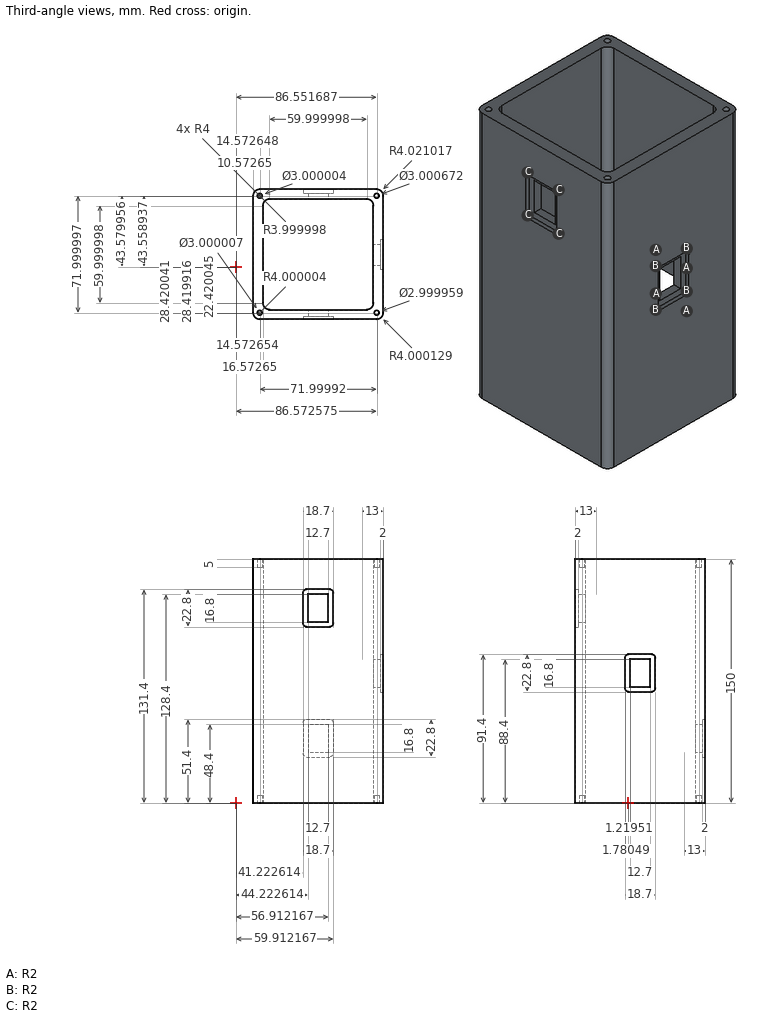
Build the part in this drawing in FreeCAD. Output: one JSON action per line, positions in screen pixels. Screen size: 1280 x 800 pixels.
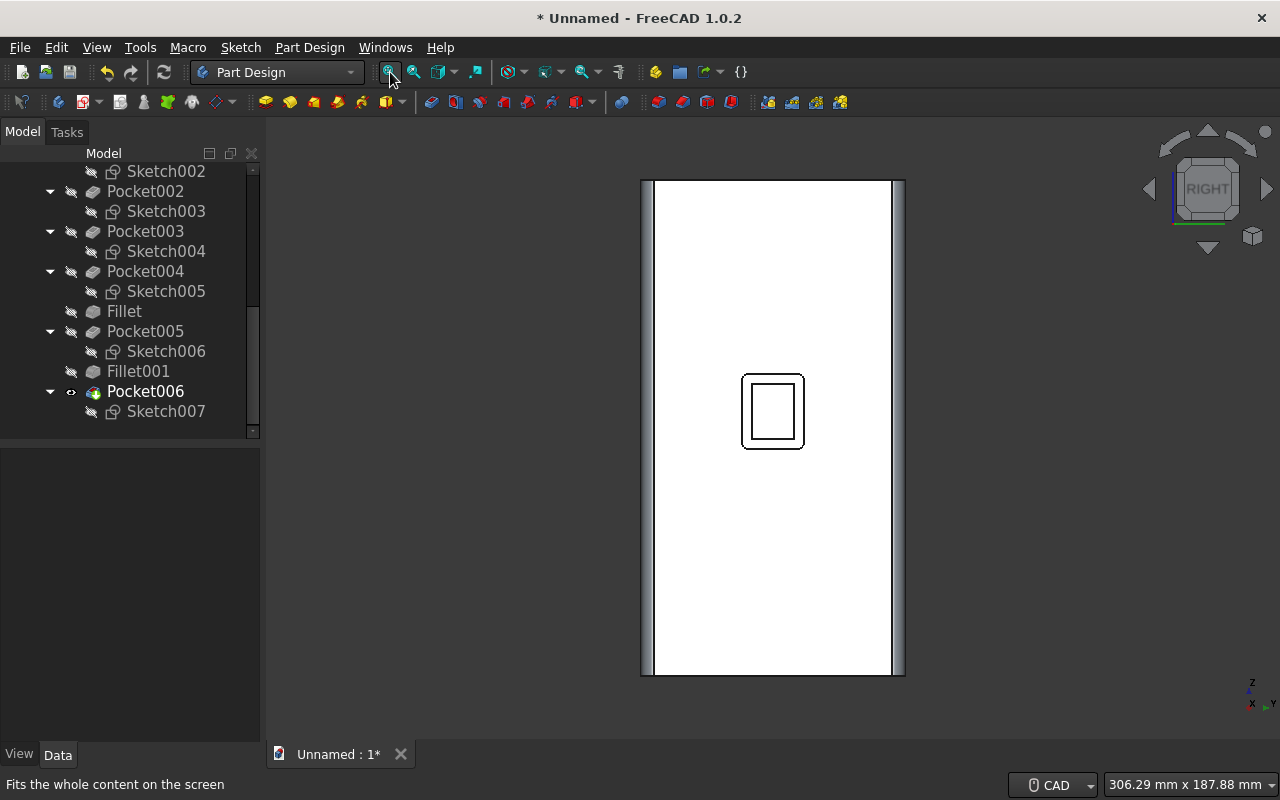
{"action": "scroll", "coordinate": [644, 316], "scroll_direction": "up", "scroll_amount": 9}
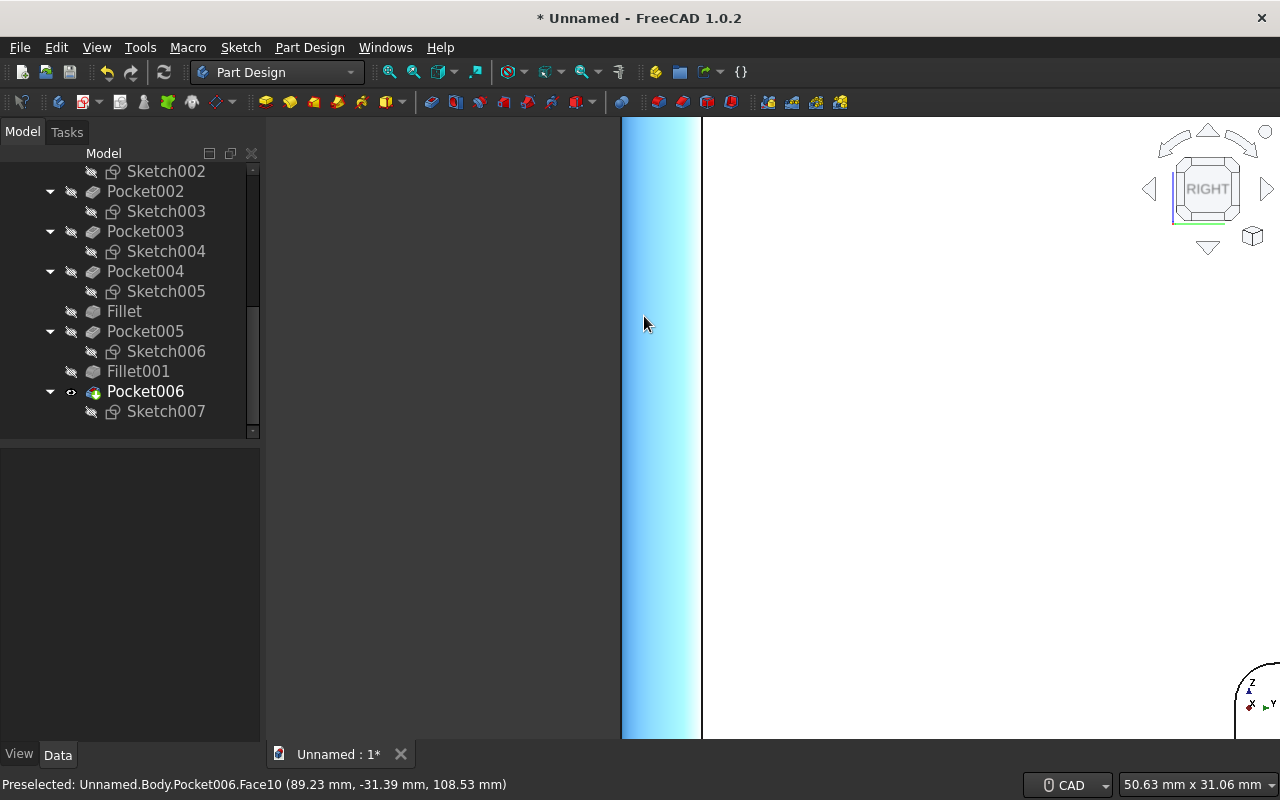
{"action": "left_click", "coordinate": [390, 72]}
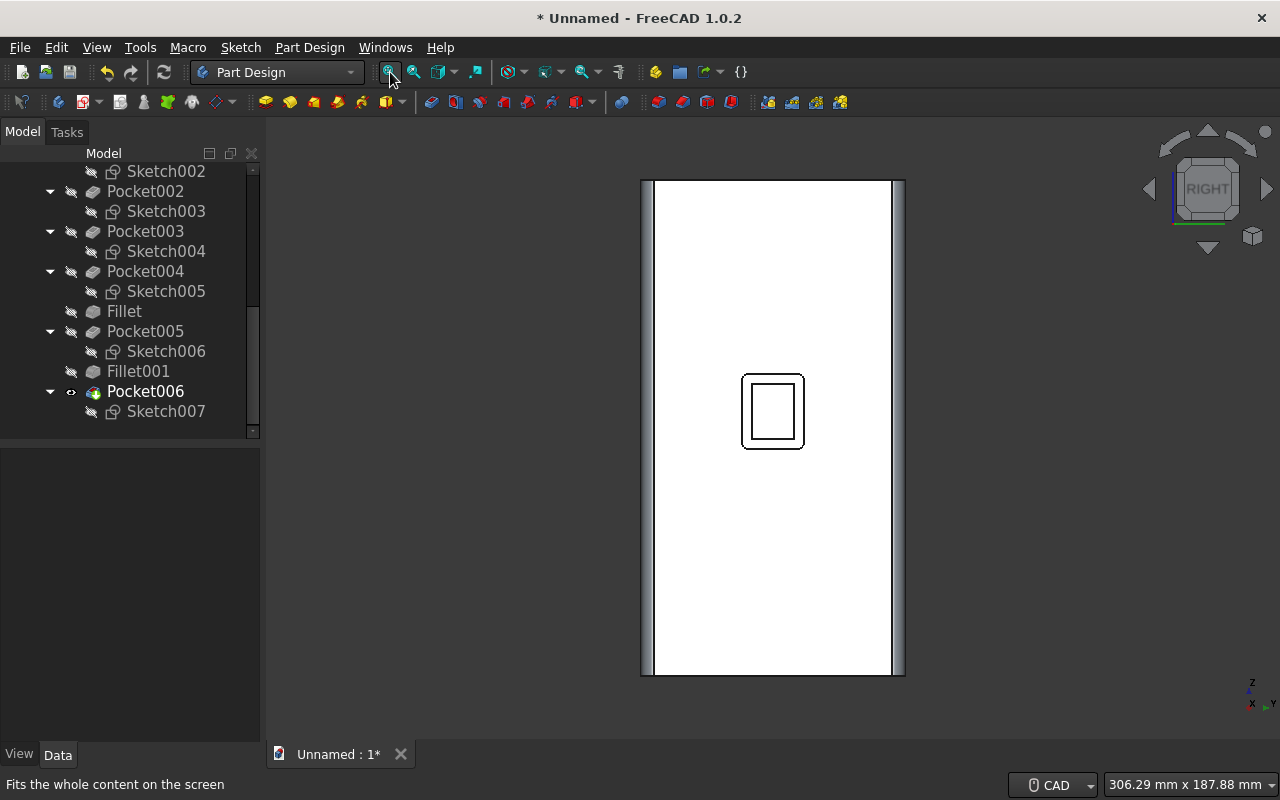
{"action": "key", "text": "5"}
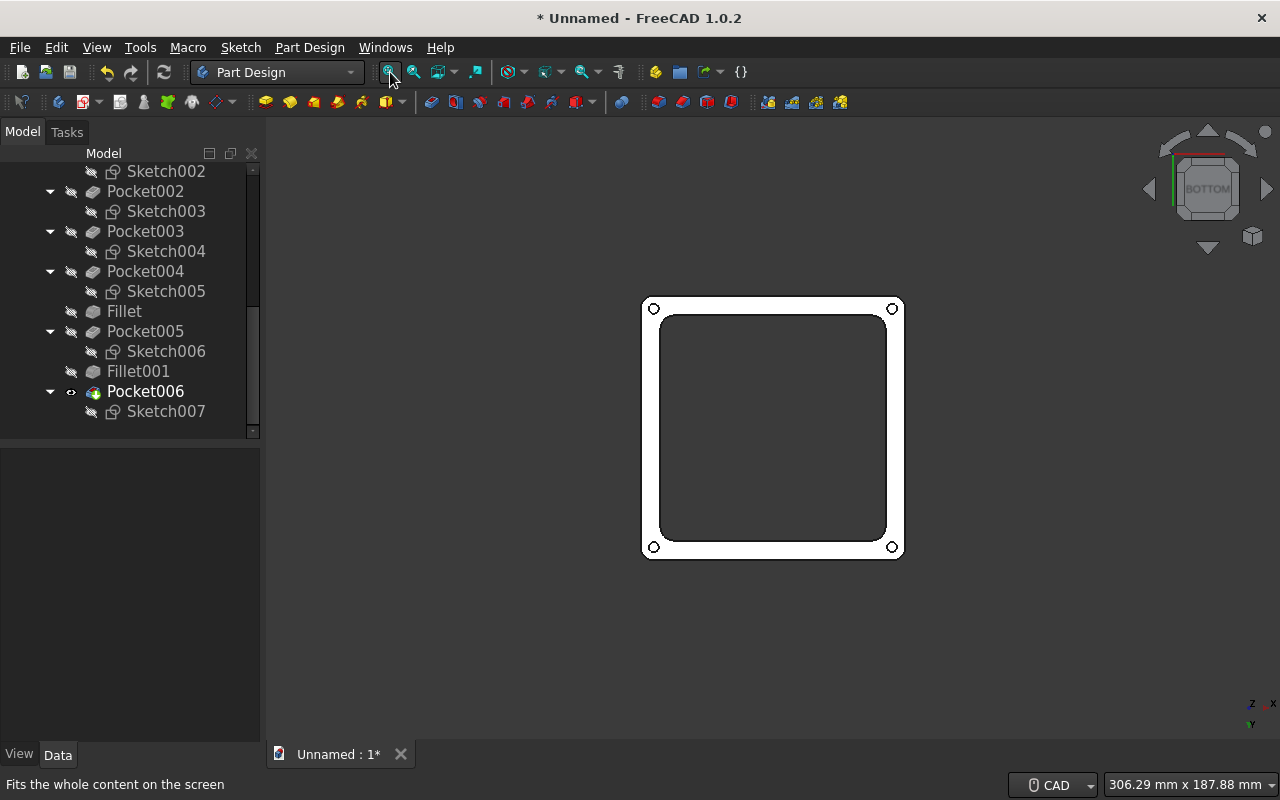
{"action": "left_click", "coordinate": [390, 72]}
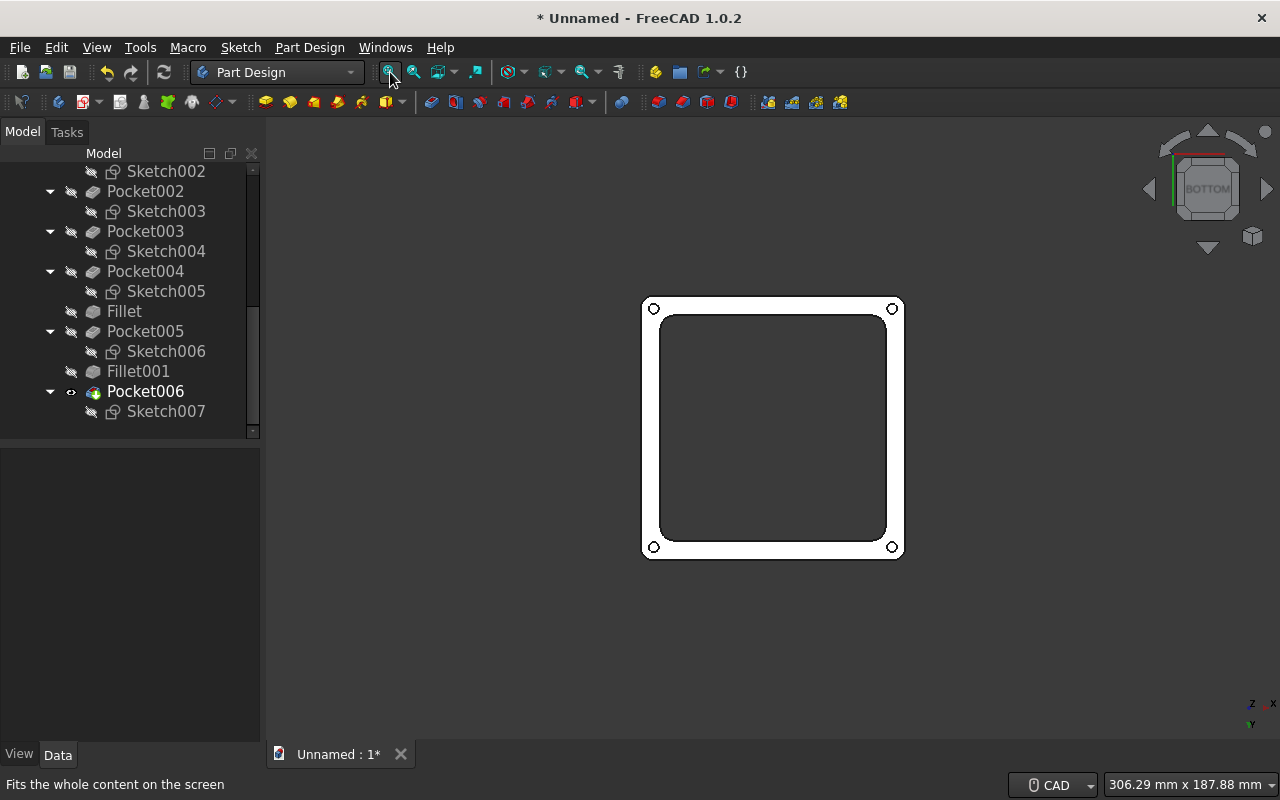
{"action": "scroll", "coordinate": [742, 298], "scroll_direction": "up", "scroll_amount": 9}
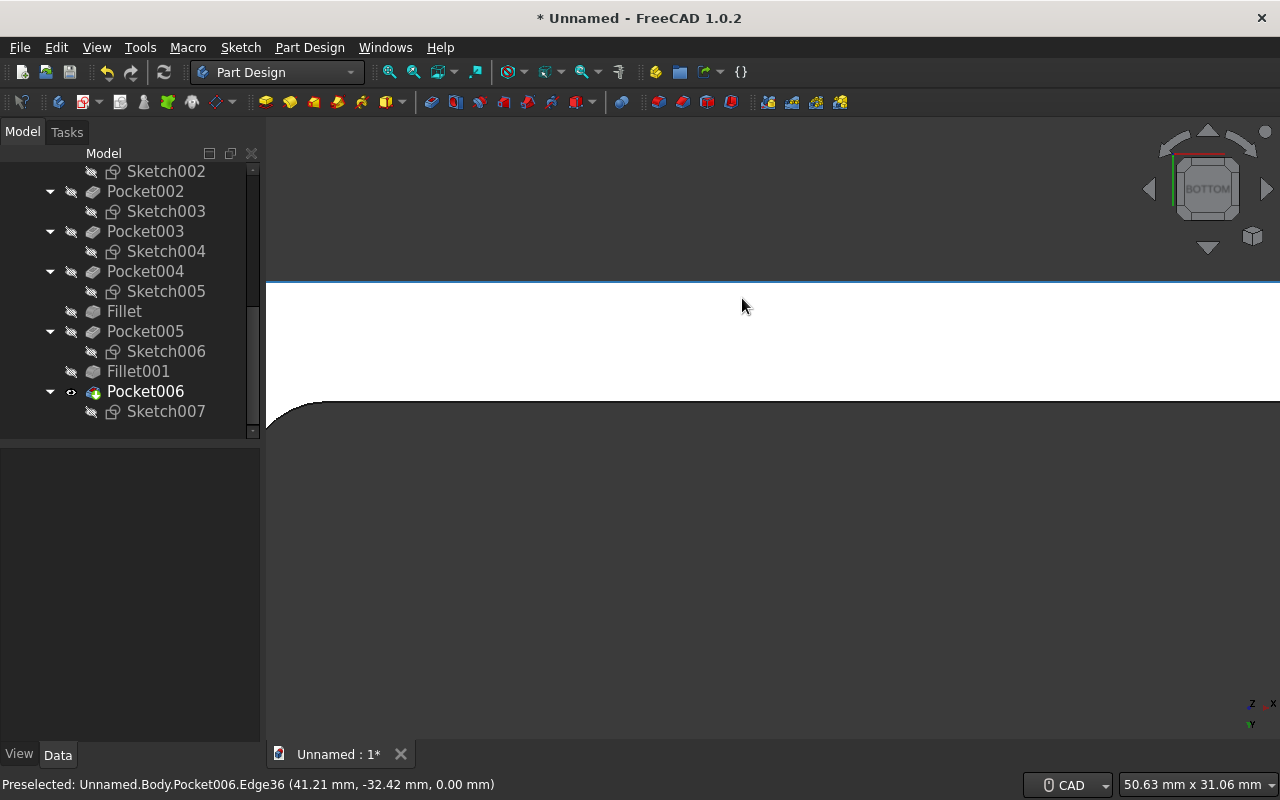
{"action": "left_click", "coordinate": [390, 72]}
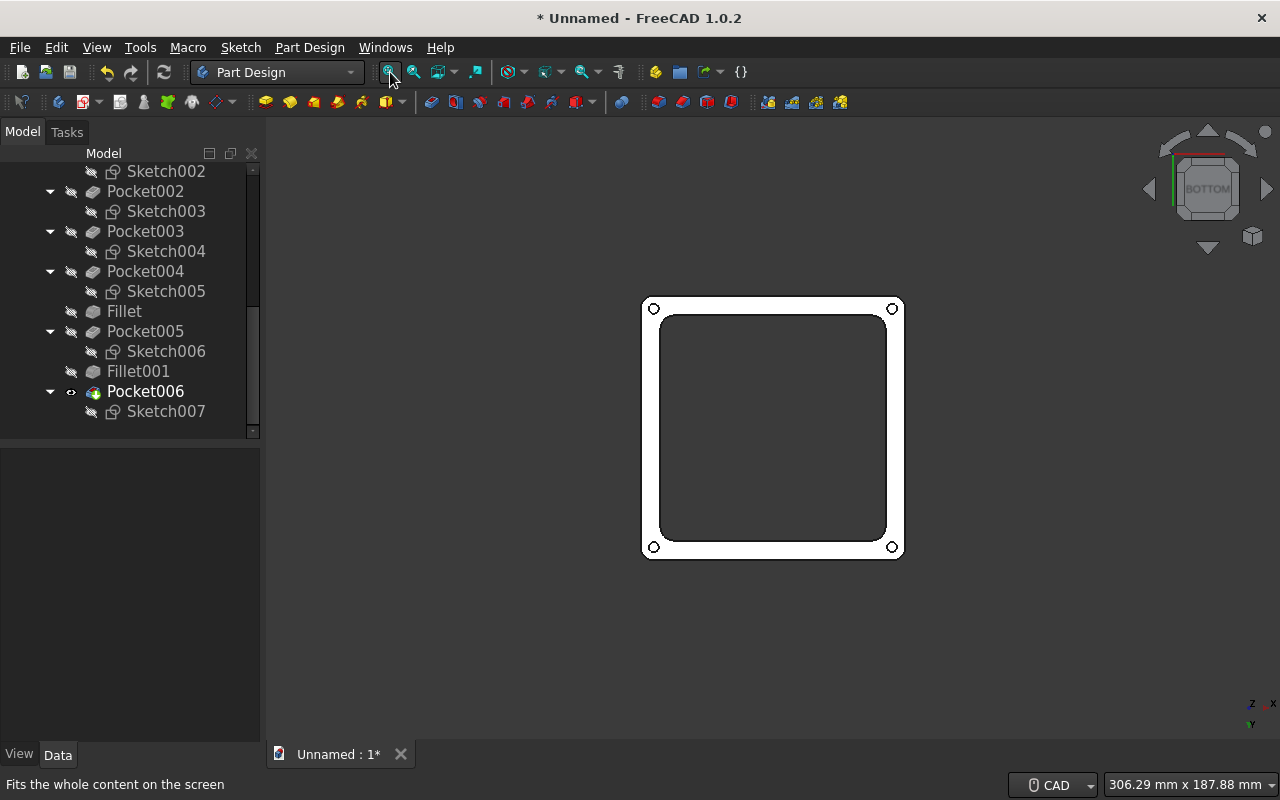
{"action": "key", "text": "4"}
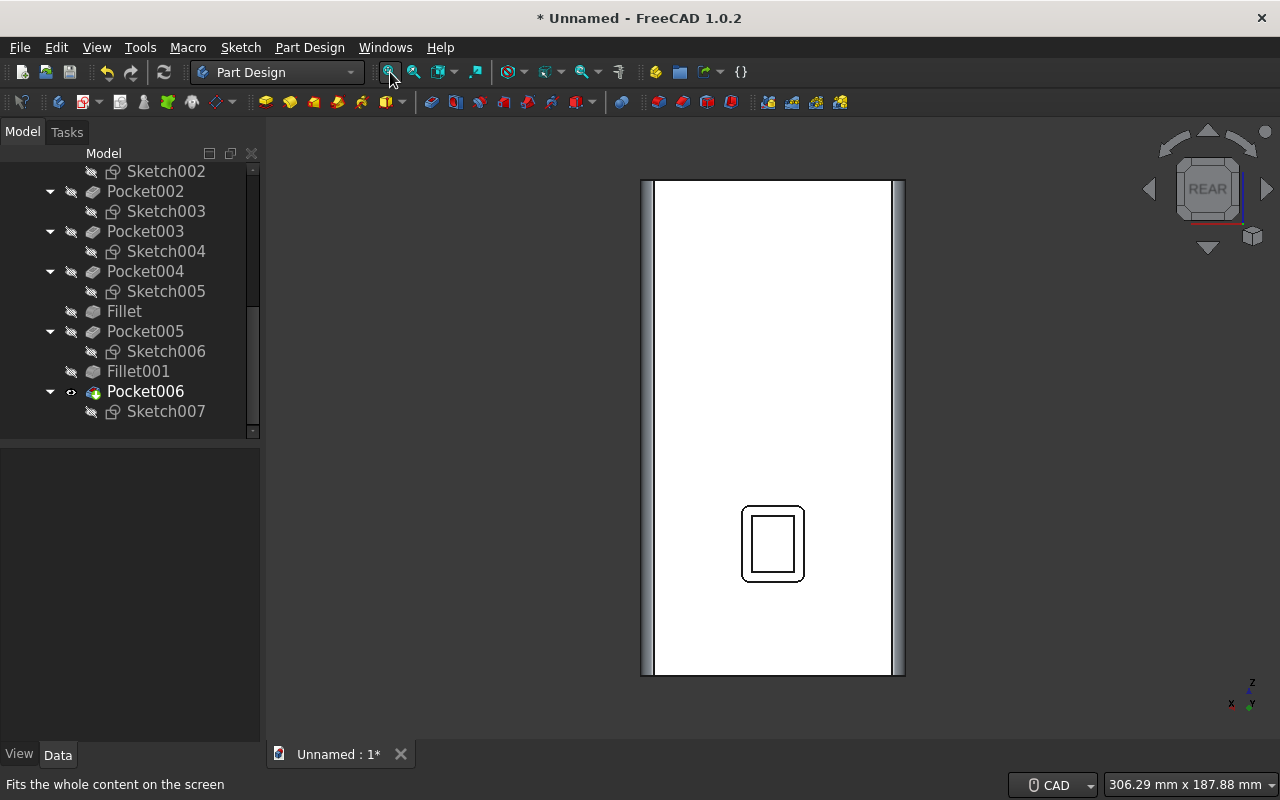
{"action": "scroll", "coordinate": [804, 316], "scroll_direction": "up", "scroll_amount": 9}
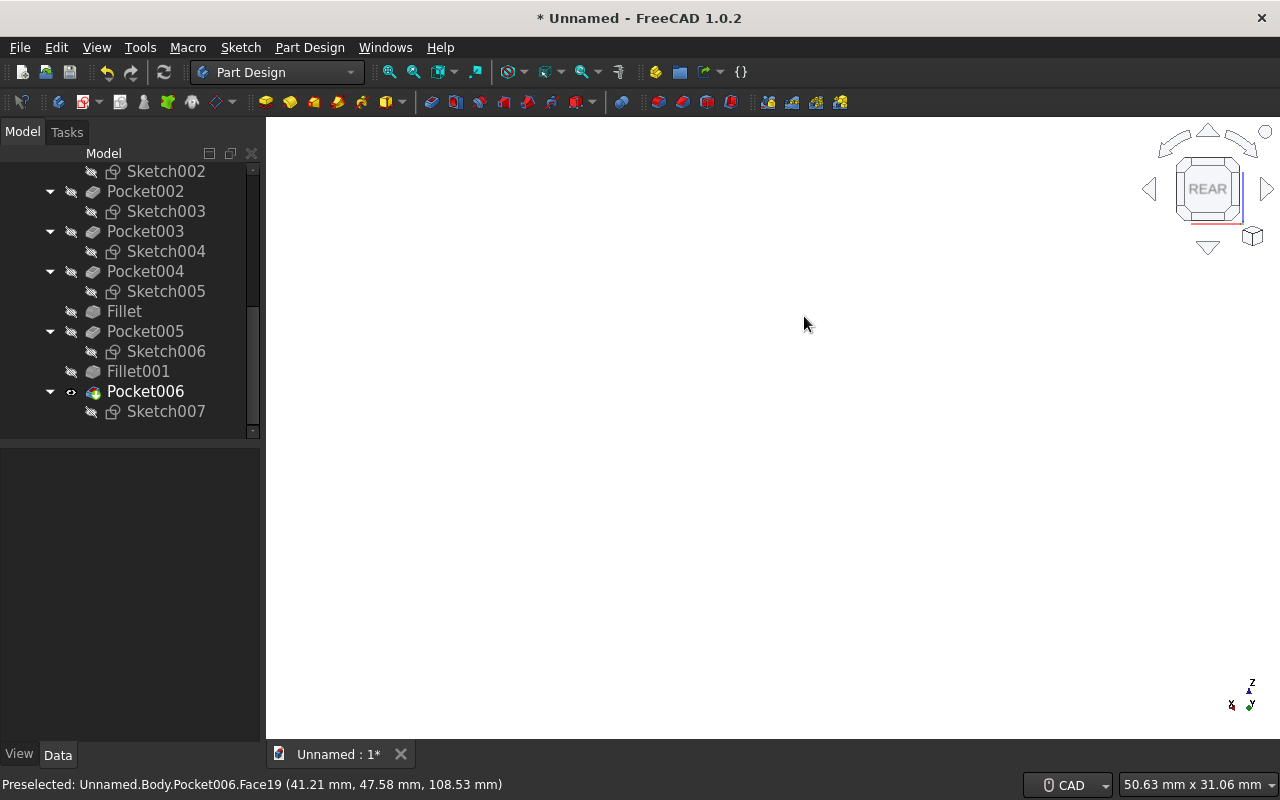
{"action": "left_click", "coordinate": [390, 72]}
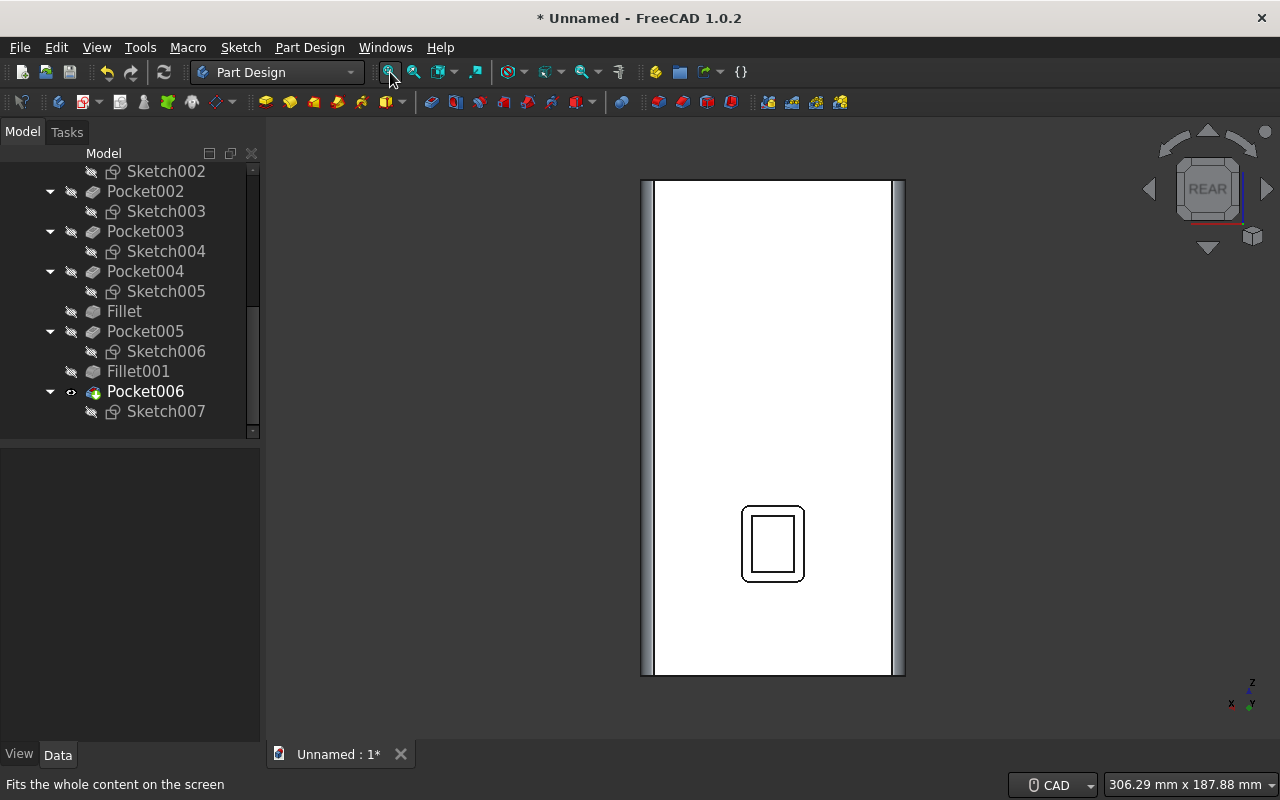
{"action": "key", "text": "6"}